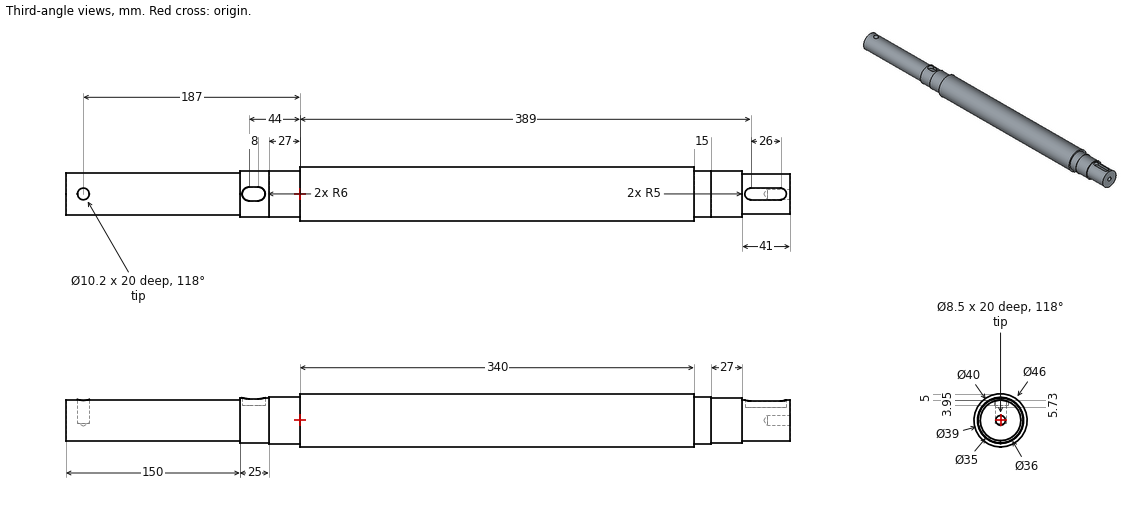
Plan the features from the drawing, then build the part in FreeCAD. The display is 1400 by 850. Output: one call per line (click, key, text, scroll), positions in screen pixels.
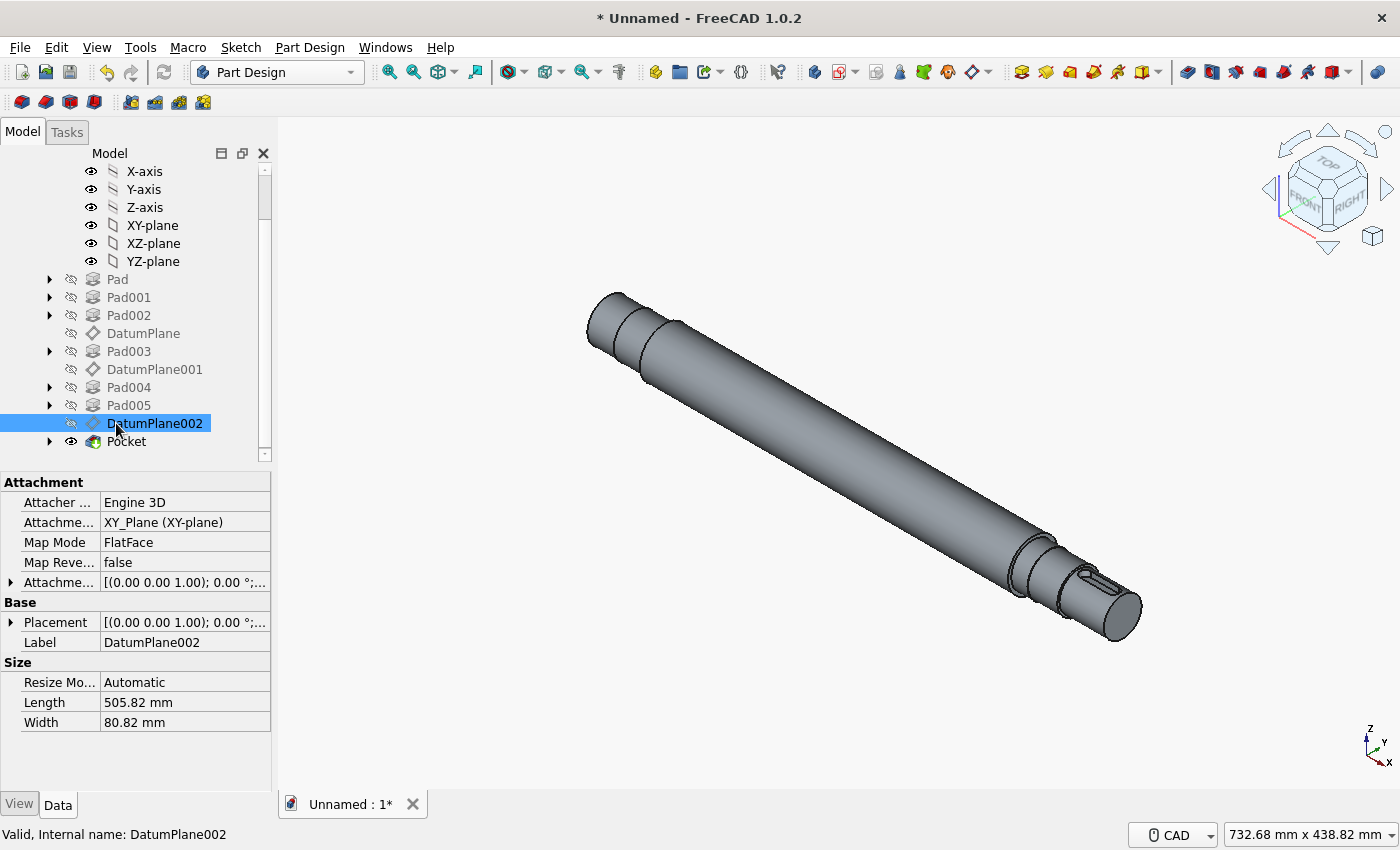
key(6)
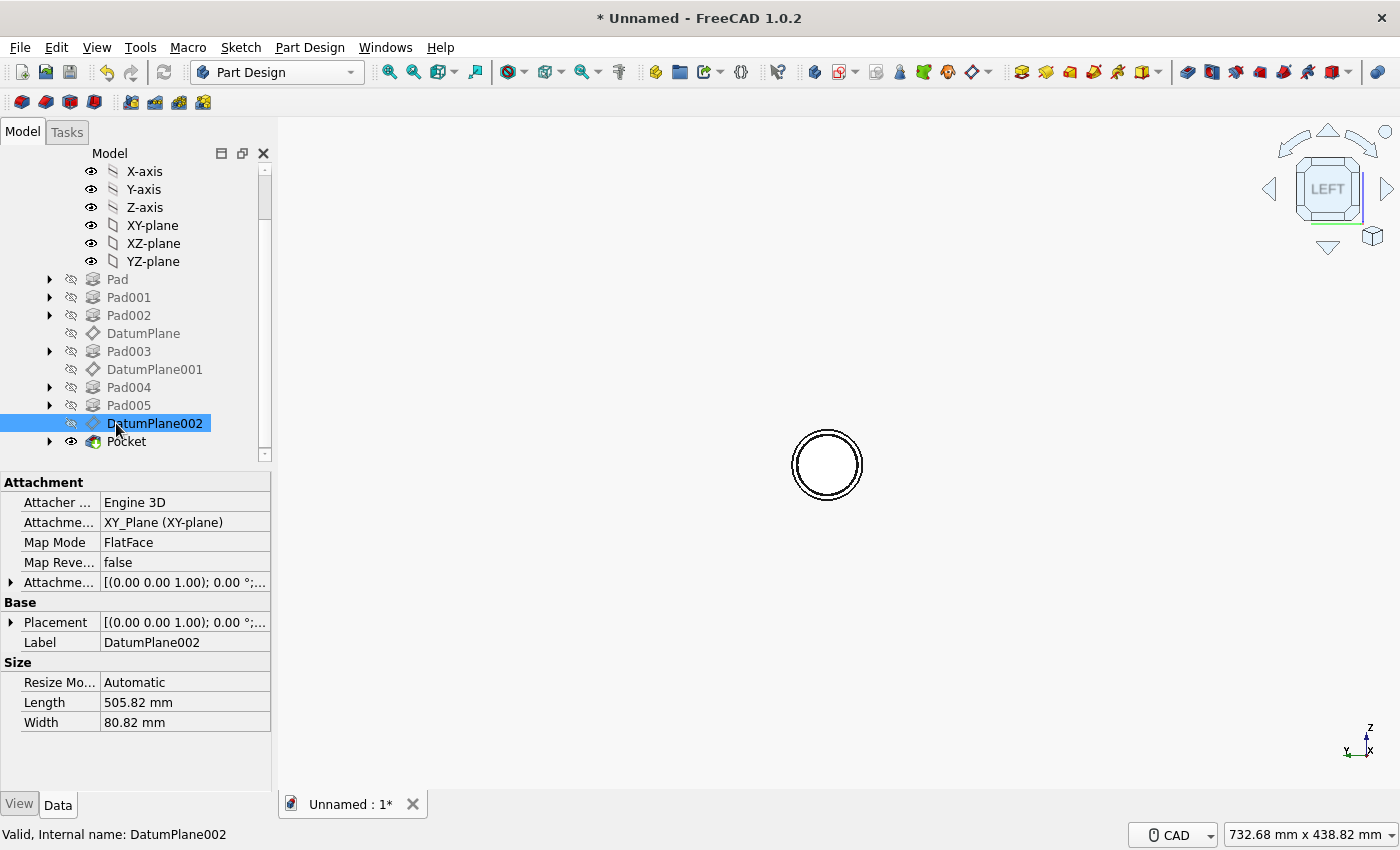
click(390, 72)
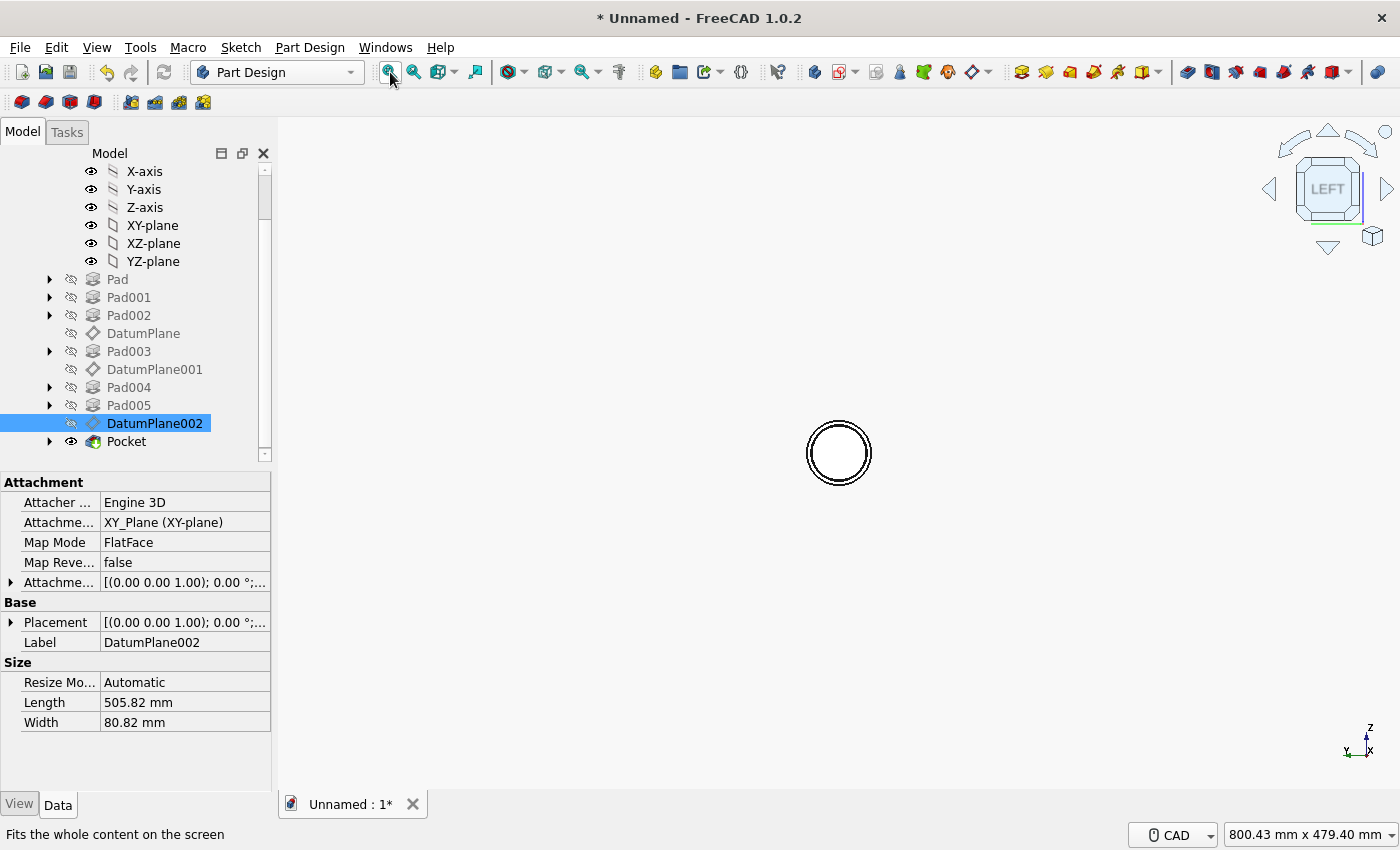
click(839, 452)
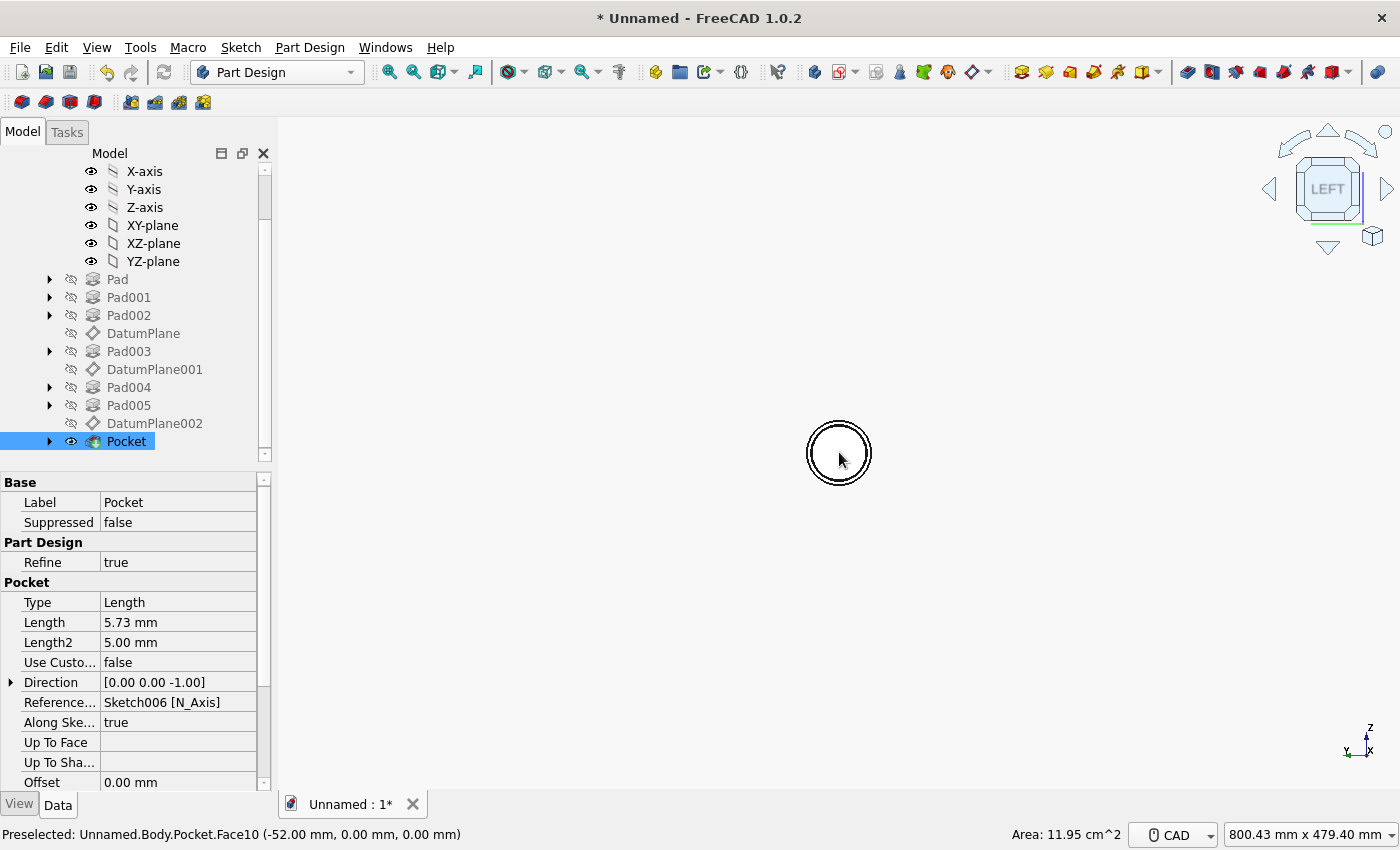
click(840, 72)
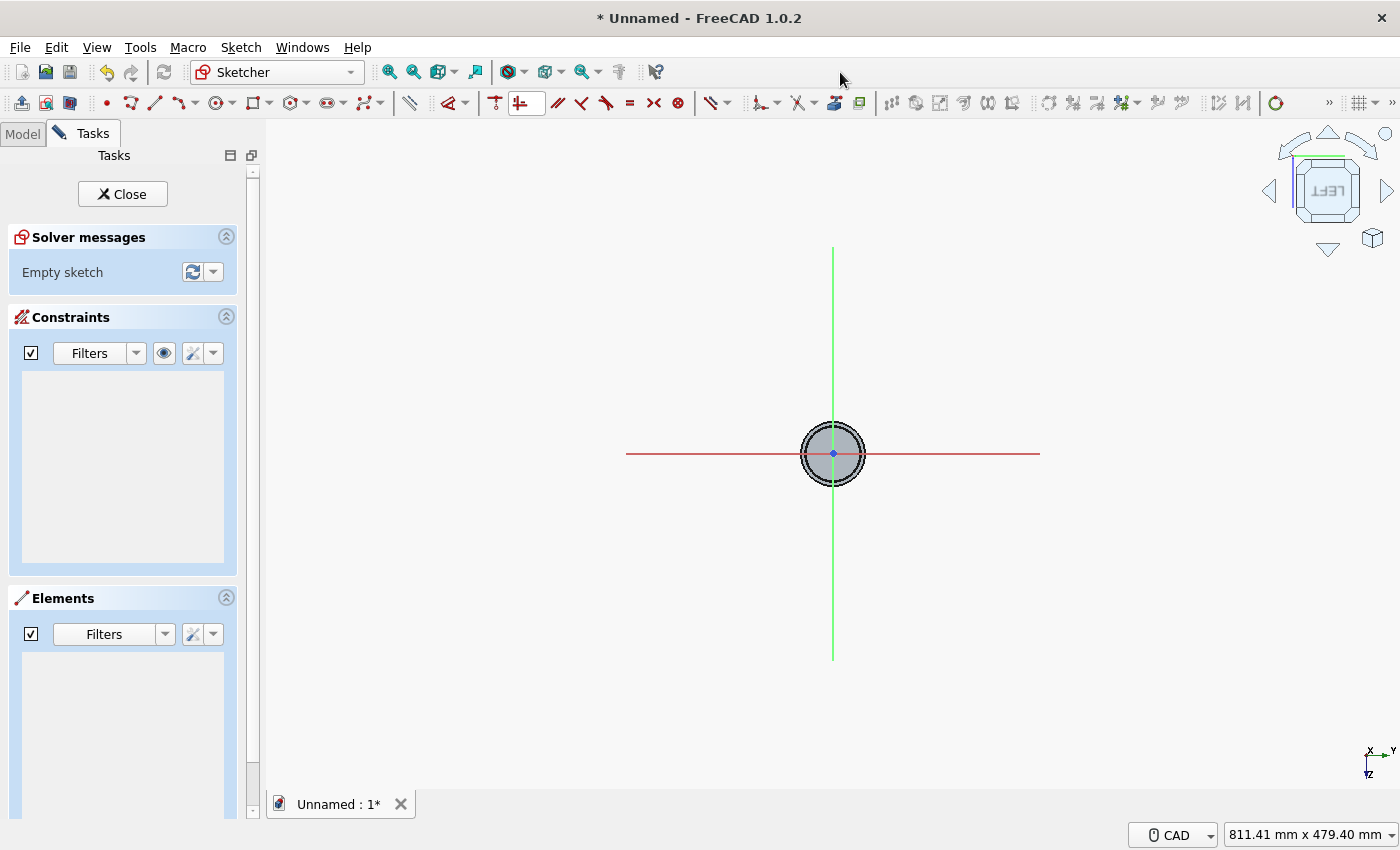
scroll(842, 454, up, 11)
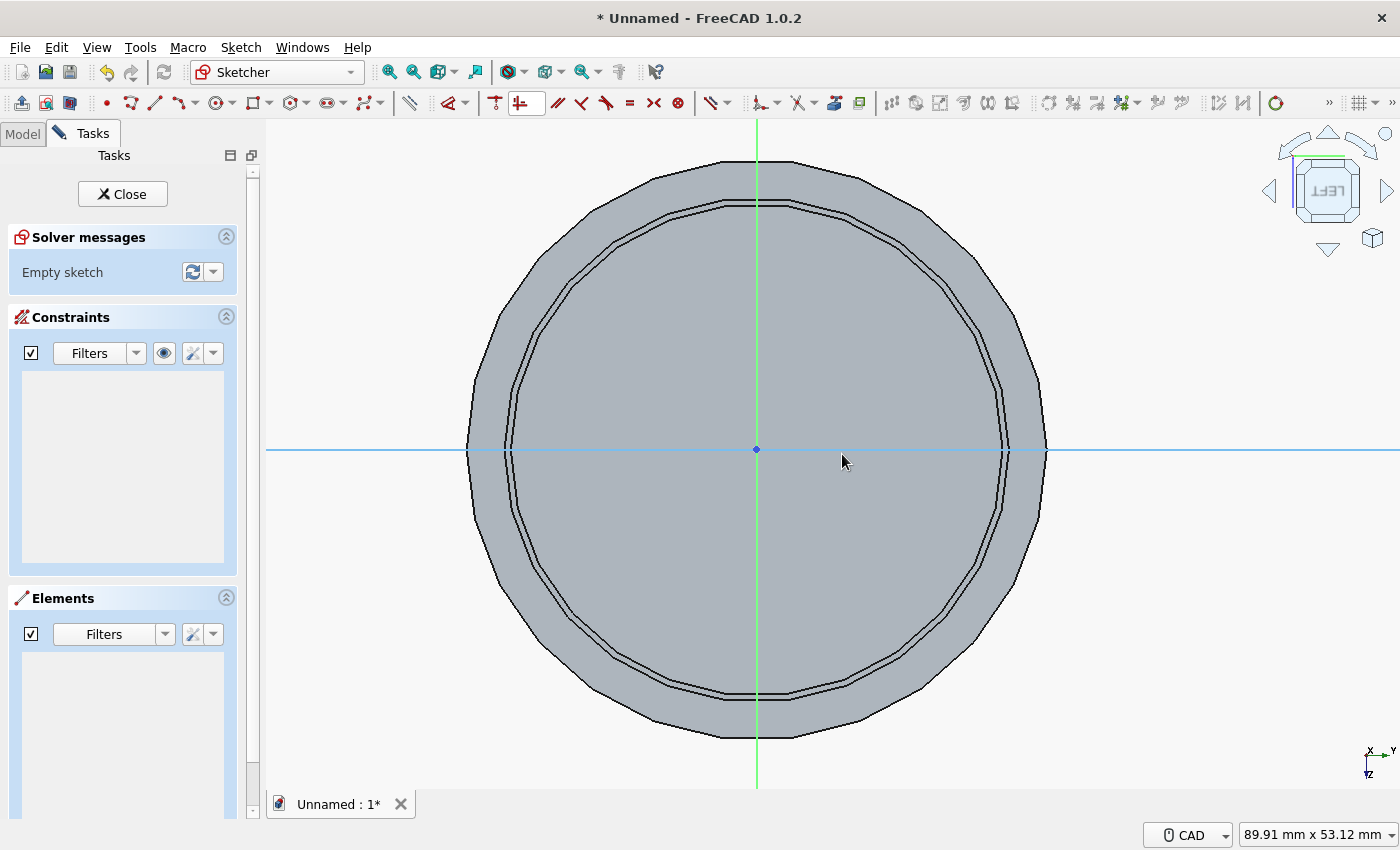
click(216, 104)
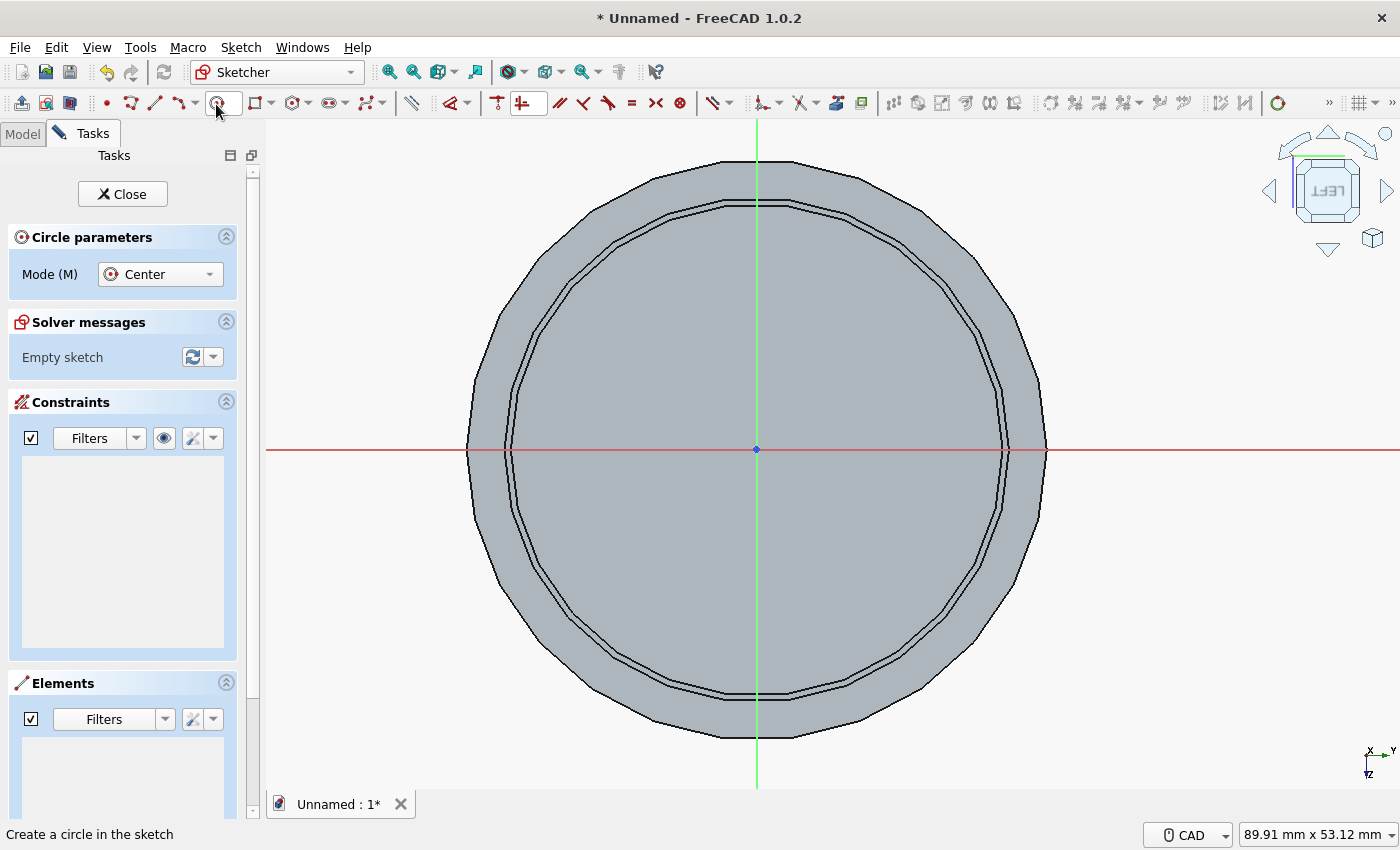
click(757, 450)
click(917, 289)
key(Escape)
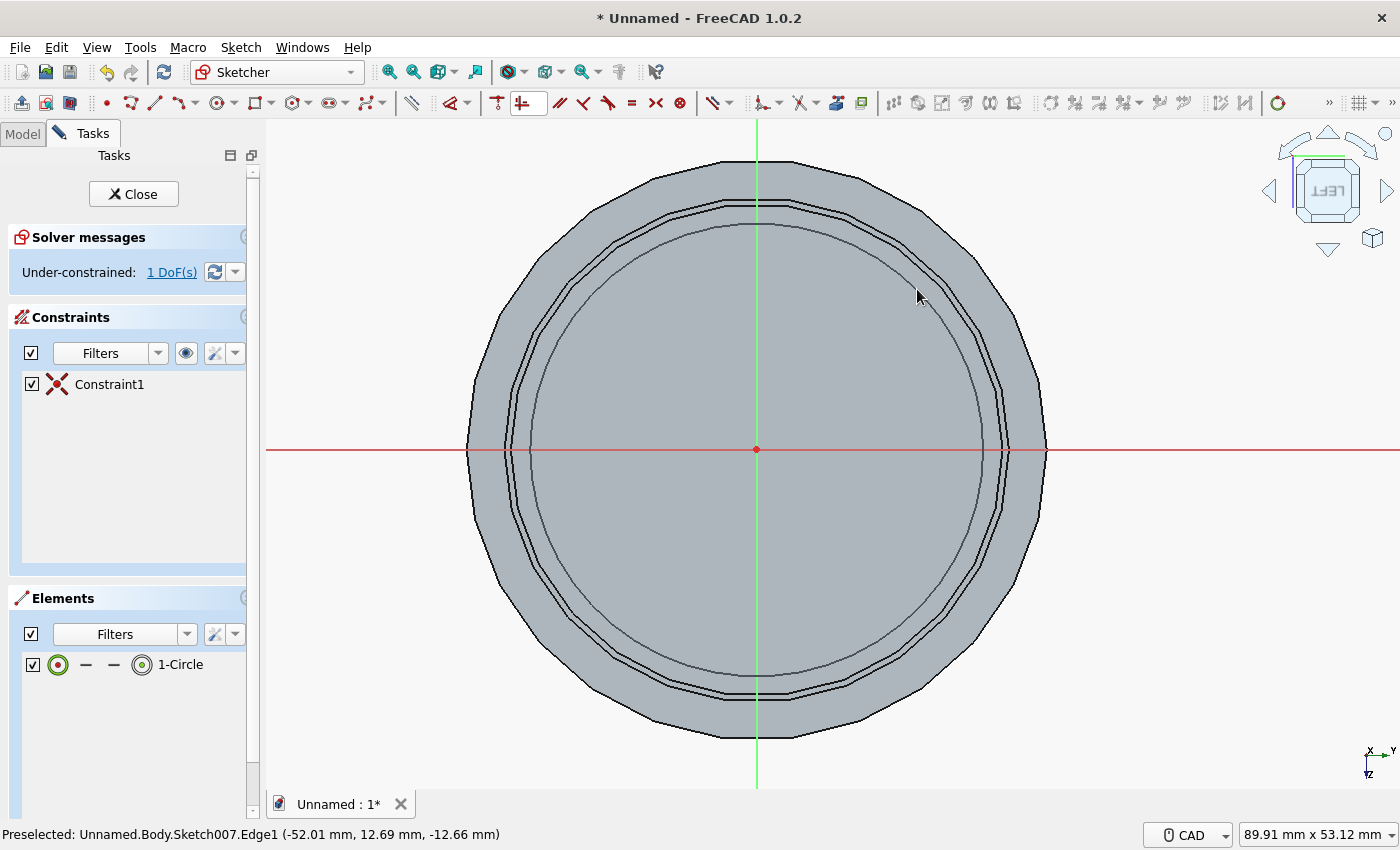
key(d)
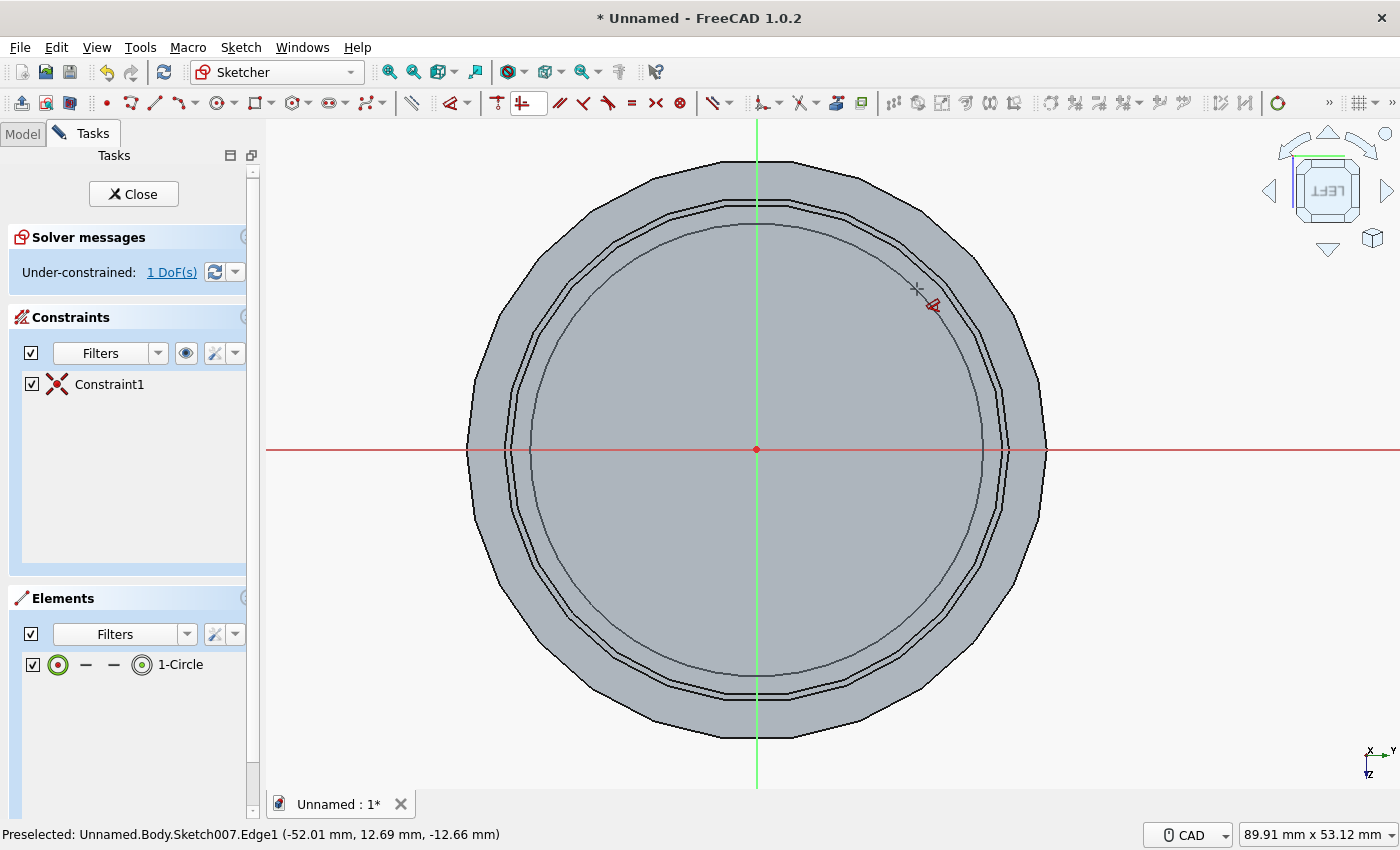
click(916, 289)
click(939, 266)